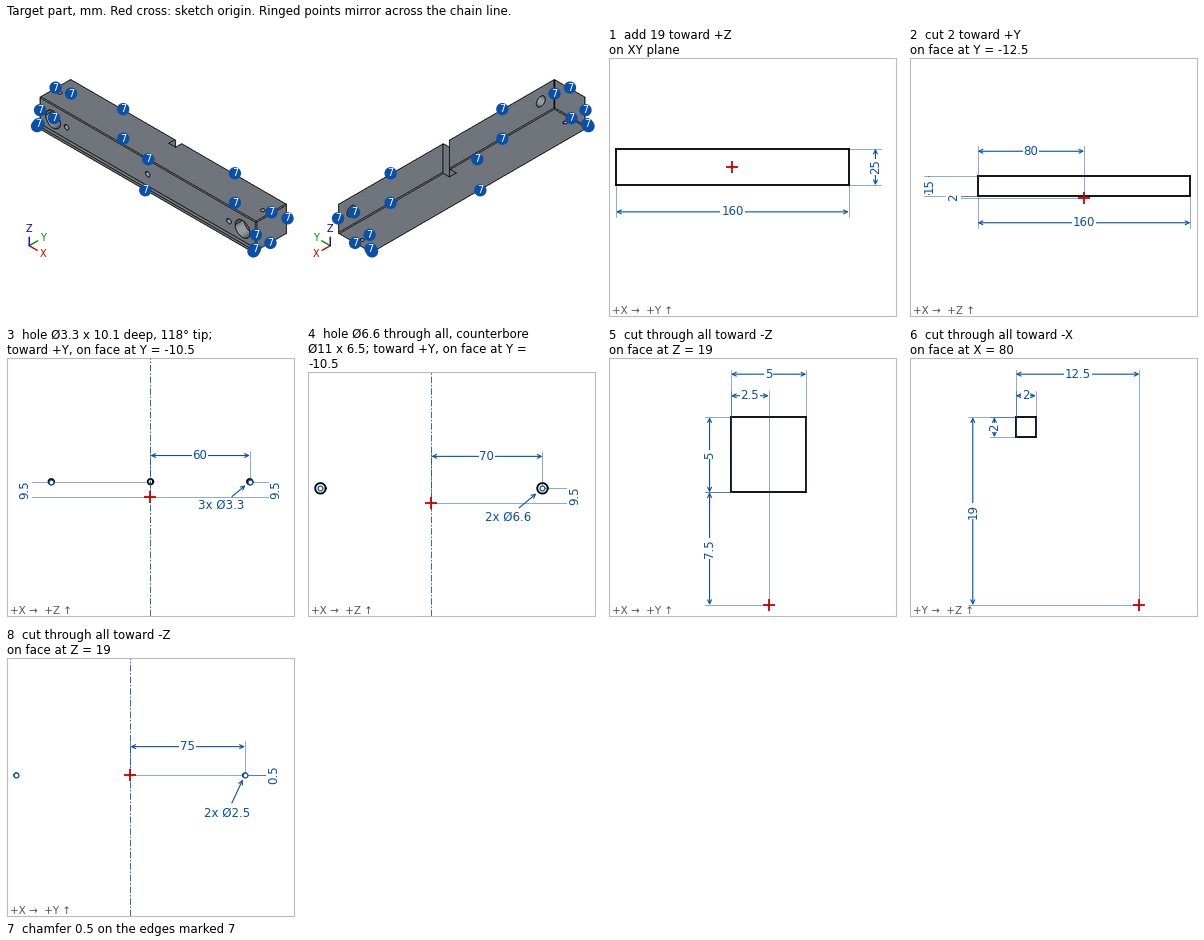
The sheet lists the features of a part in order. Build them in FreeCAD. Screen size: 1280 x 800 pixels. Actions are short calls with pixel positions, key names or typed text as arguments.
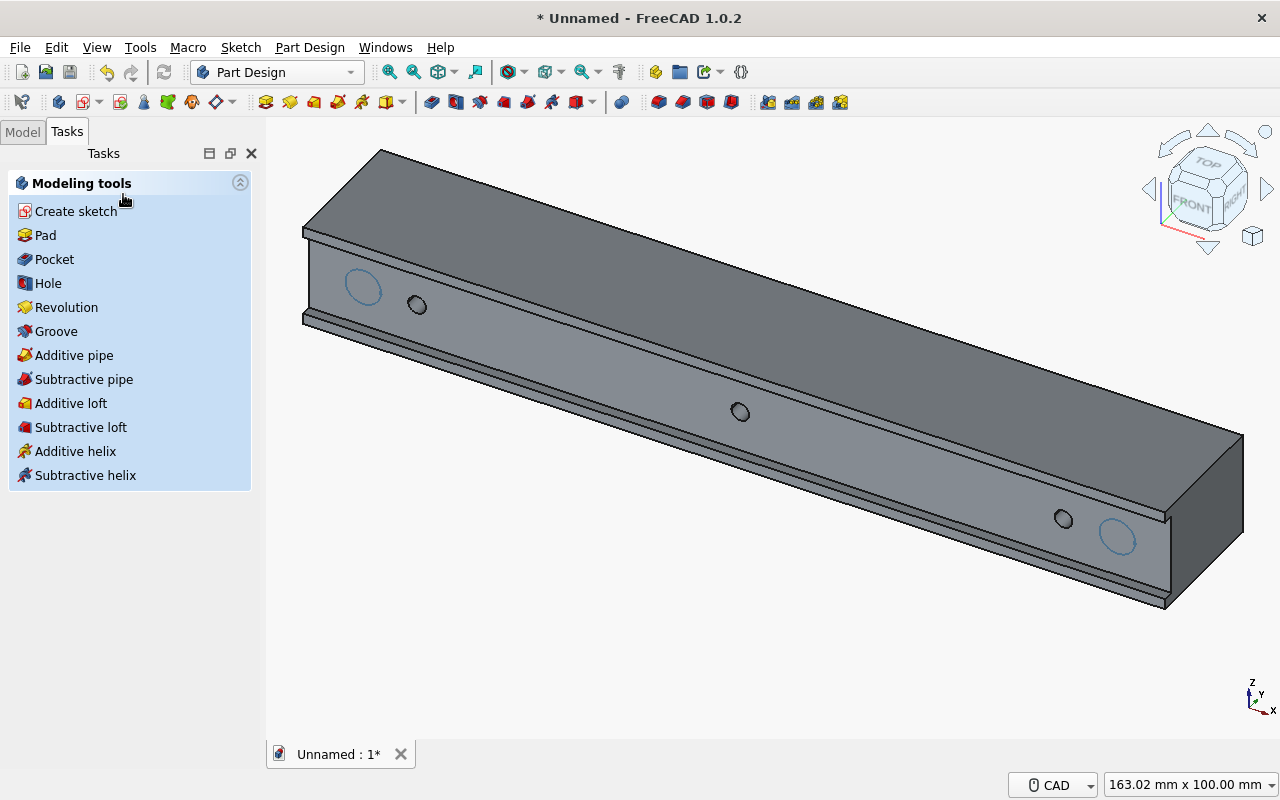
click(456, 102)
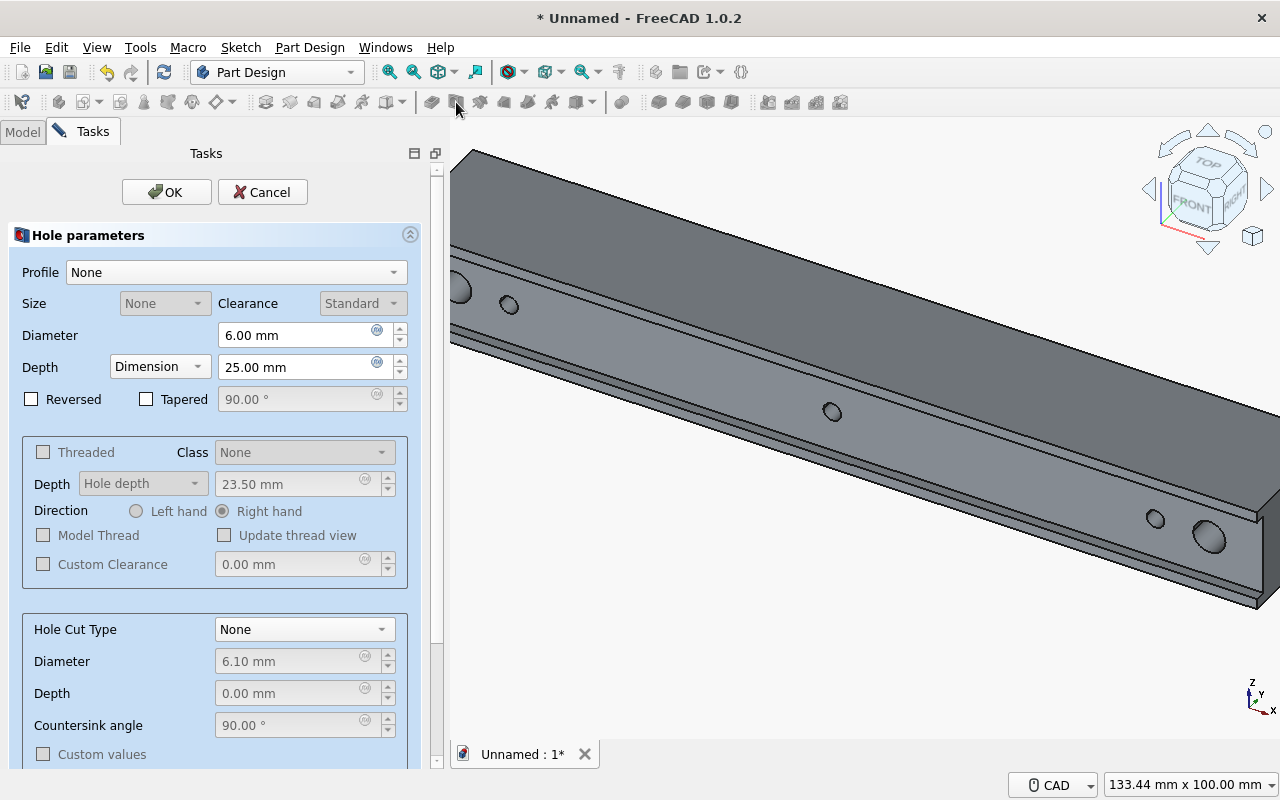
triple_click(305, 335)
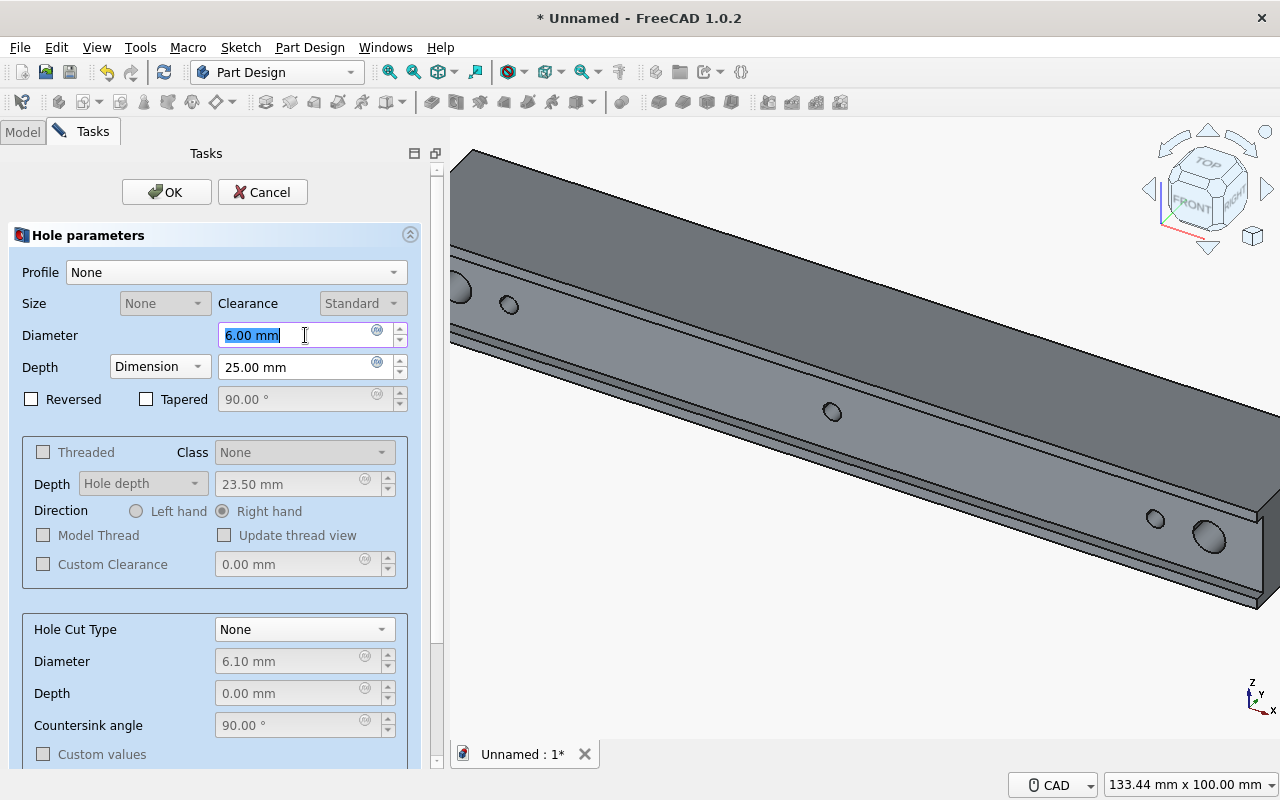
text(6.6)
key(Tab)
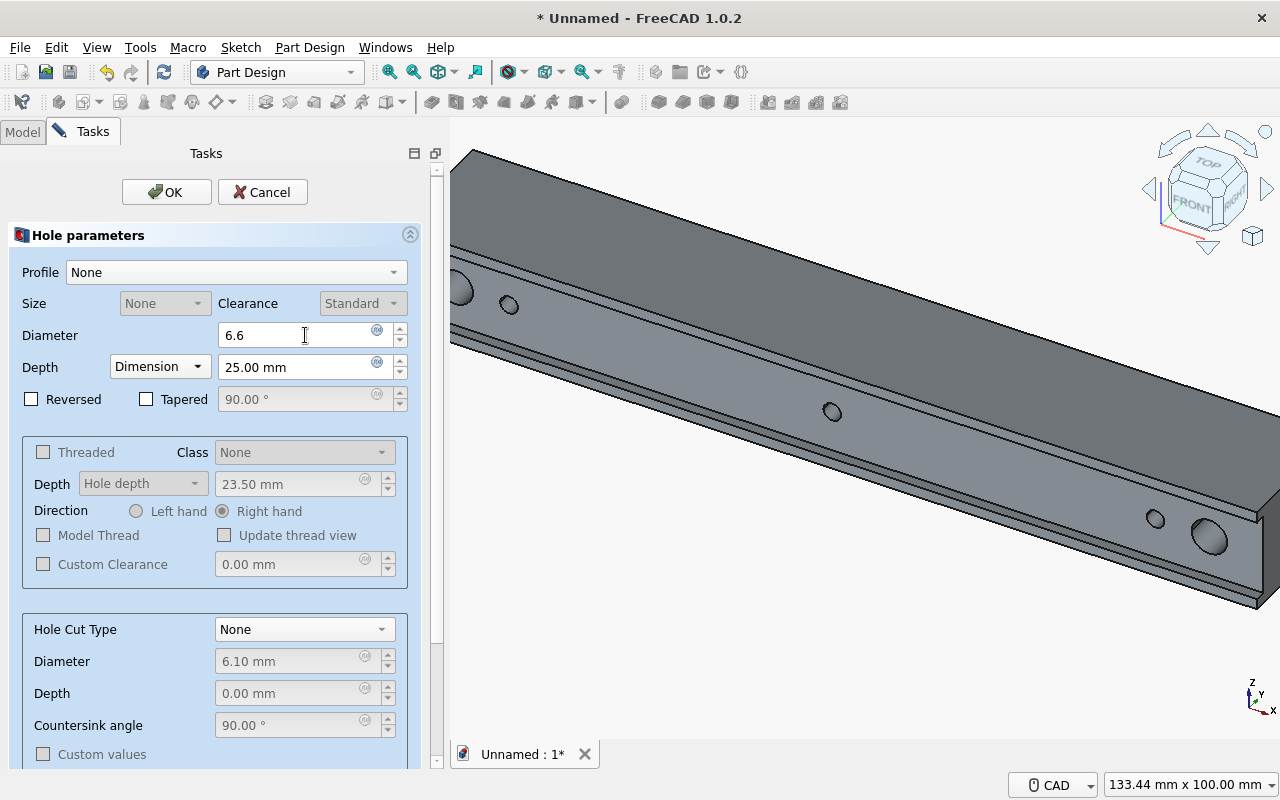
click(161, 366)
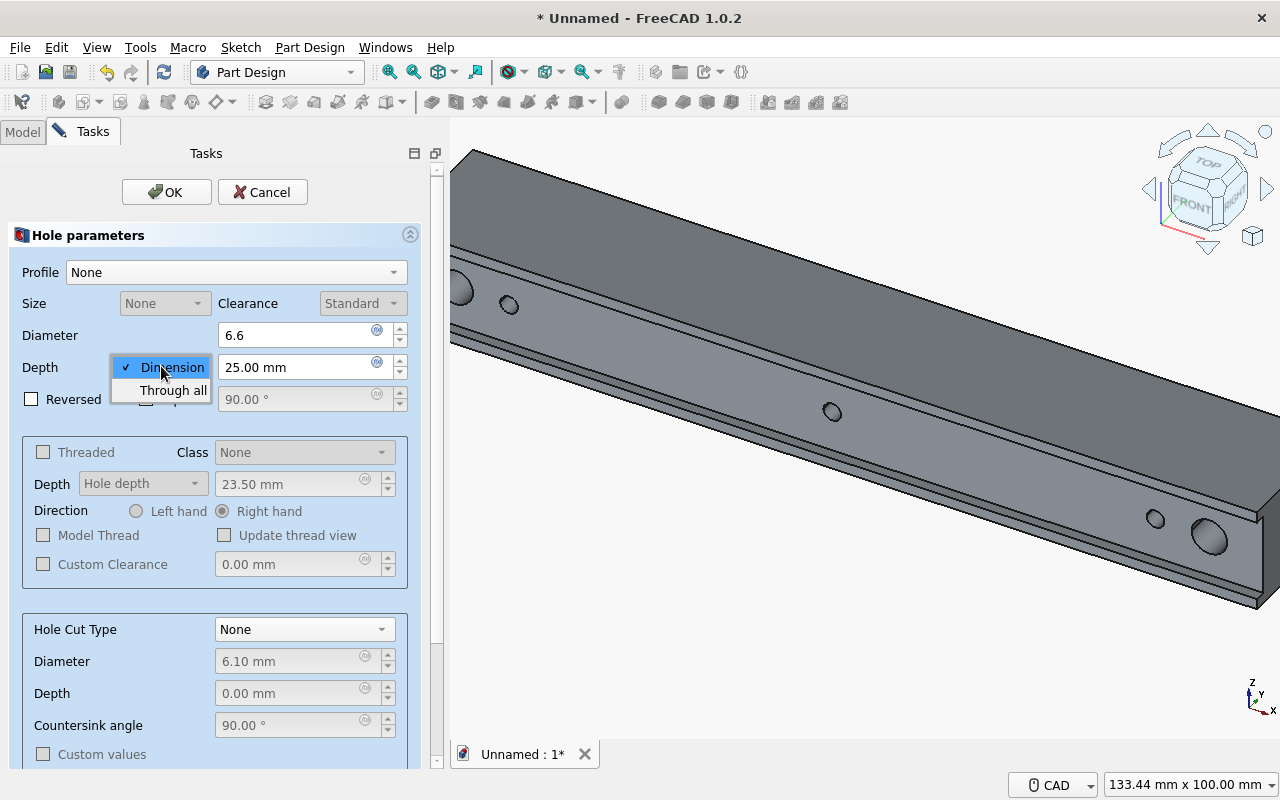
click(160, 390)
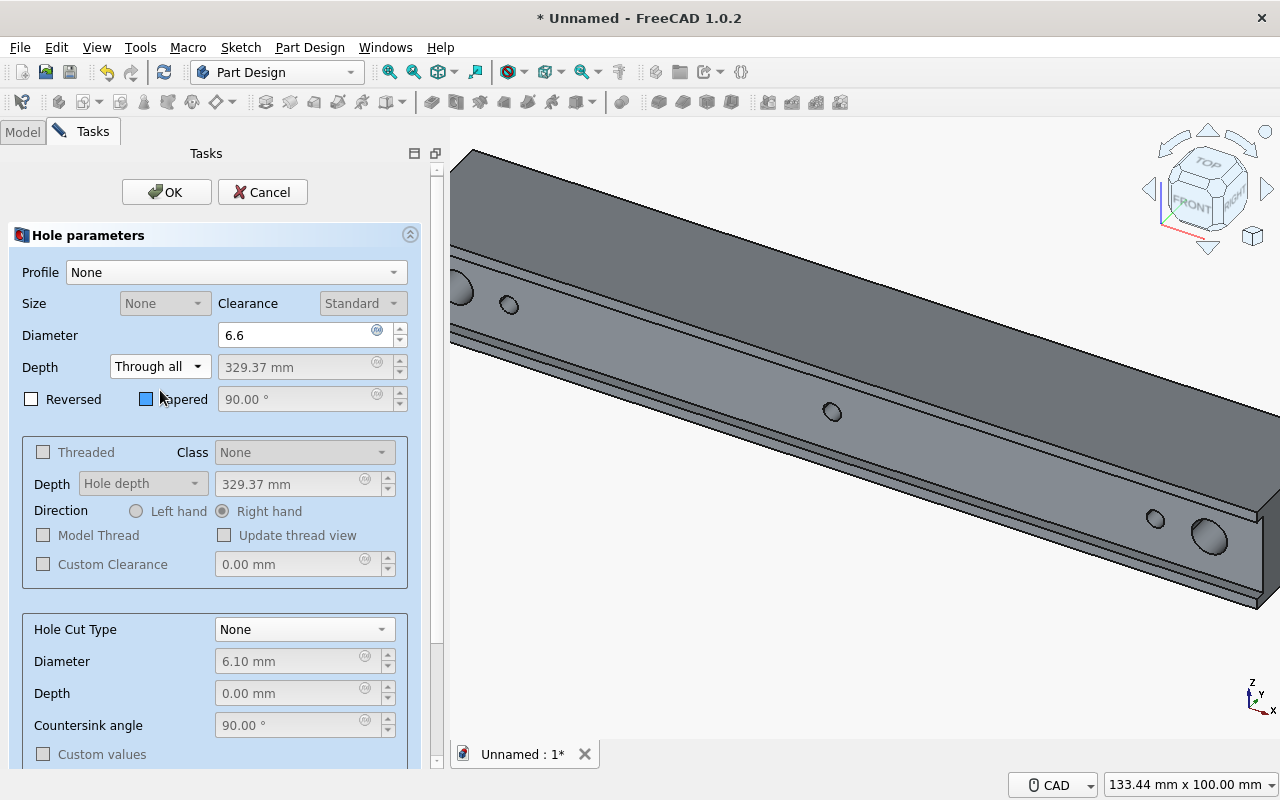
click(306, 630)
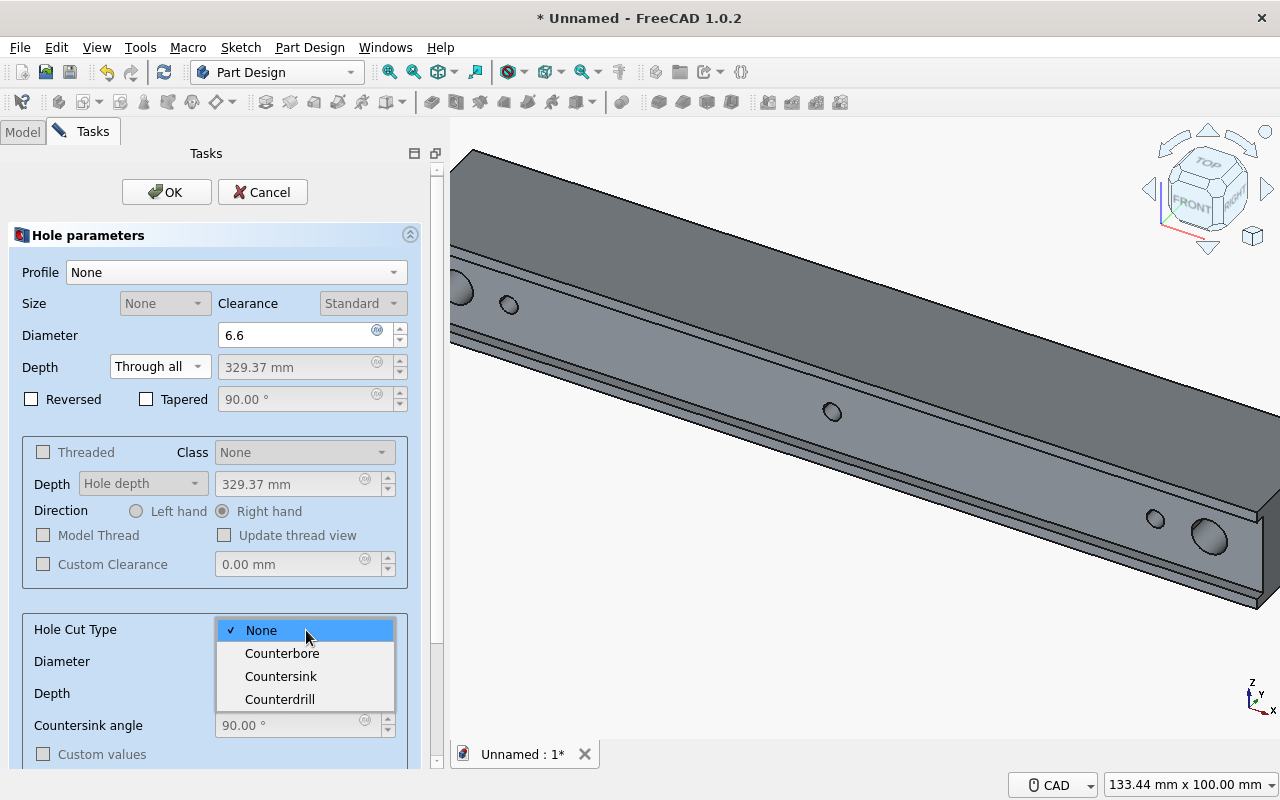
click(304, 654)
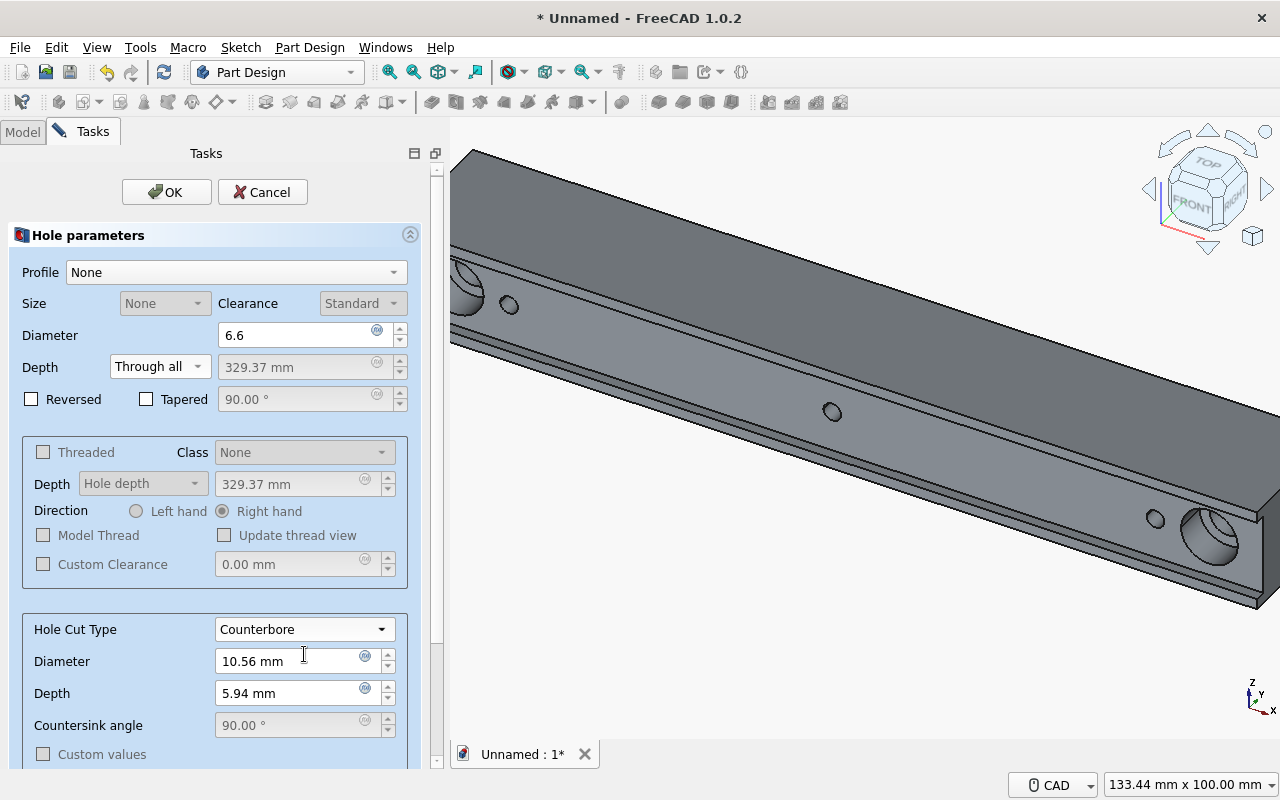
triple_click(298, 661)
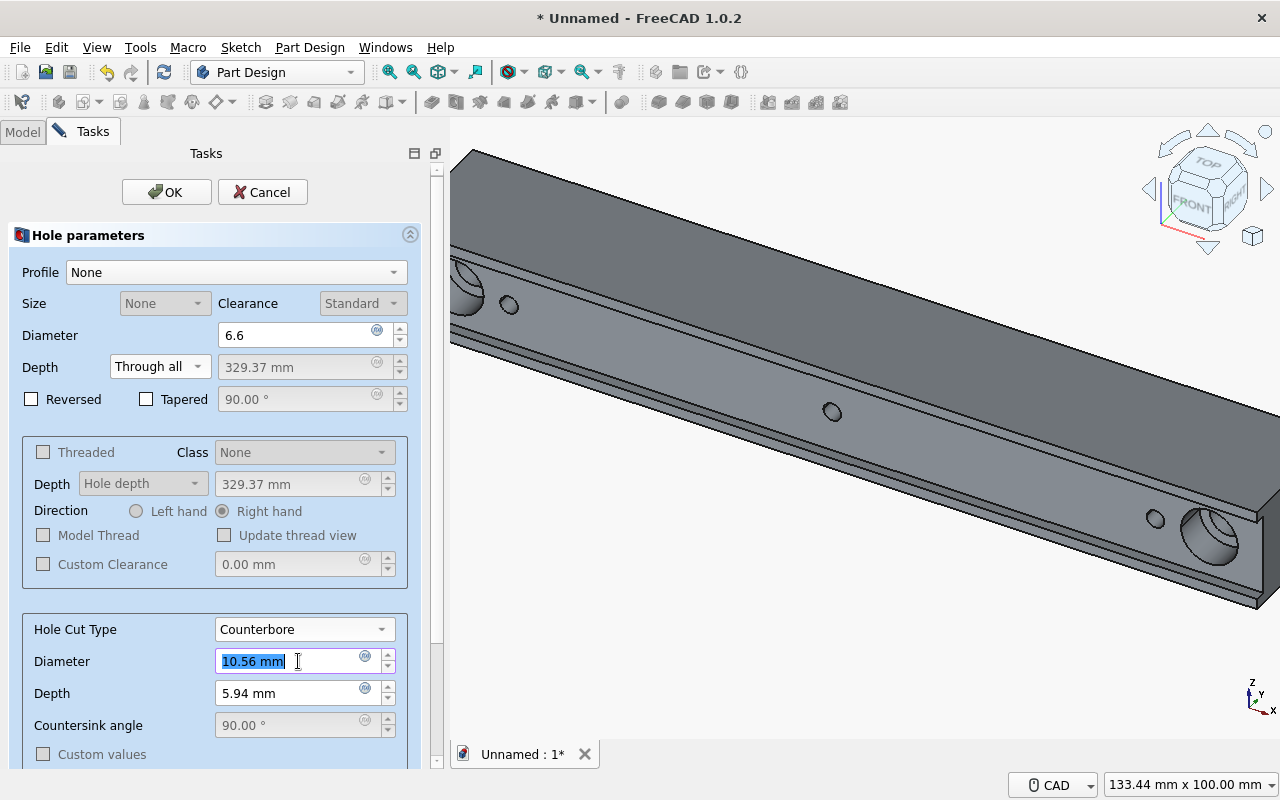
text(11)
key(Tab)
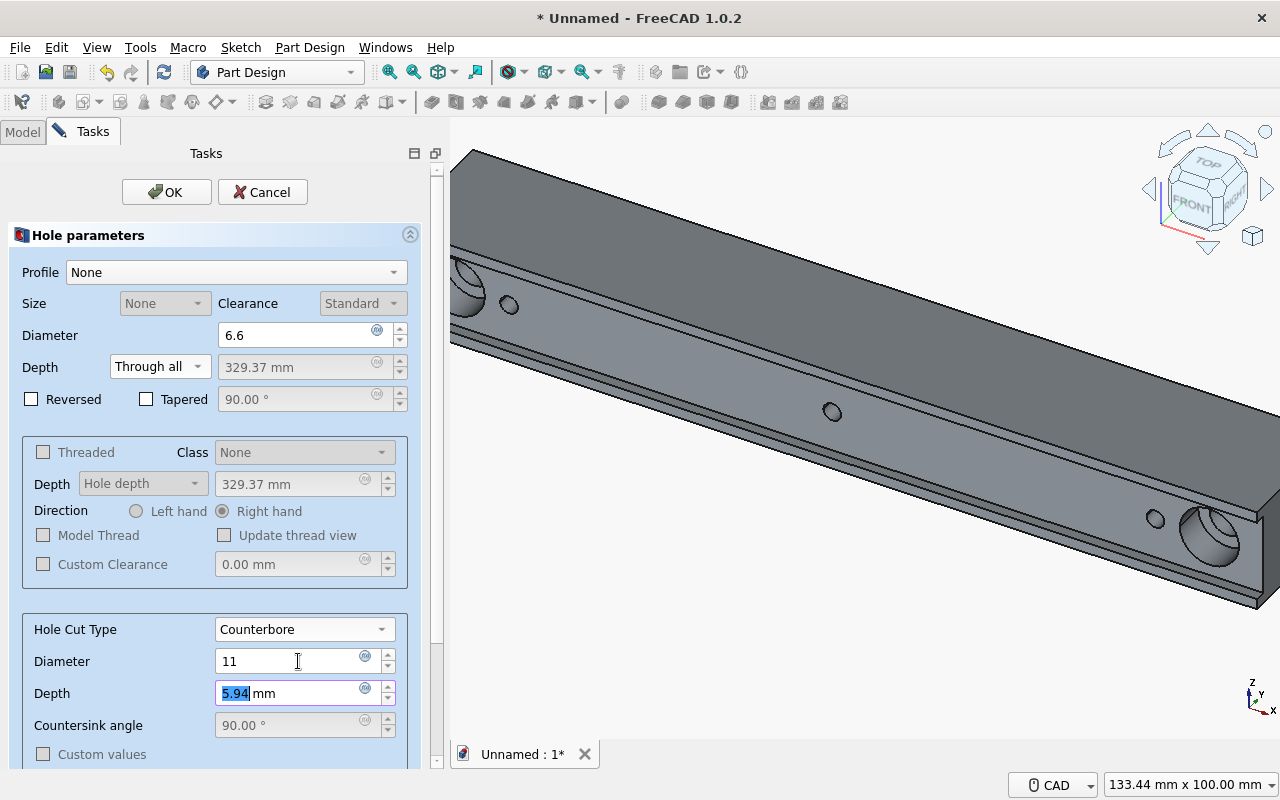
text(6.5)
key(Tab)